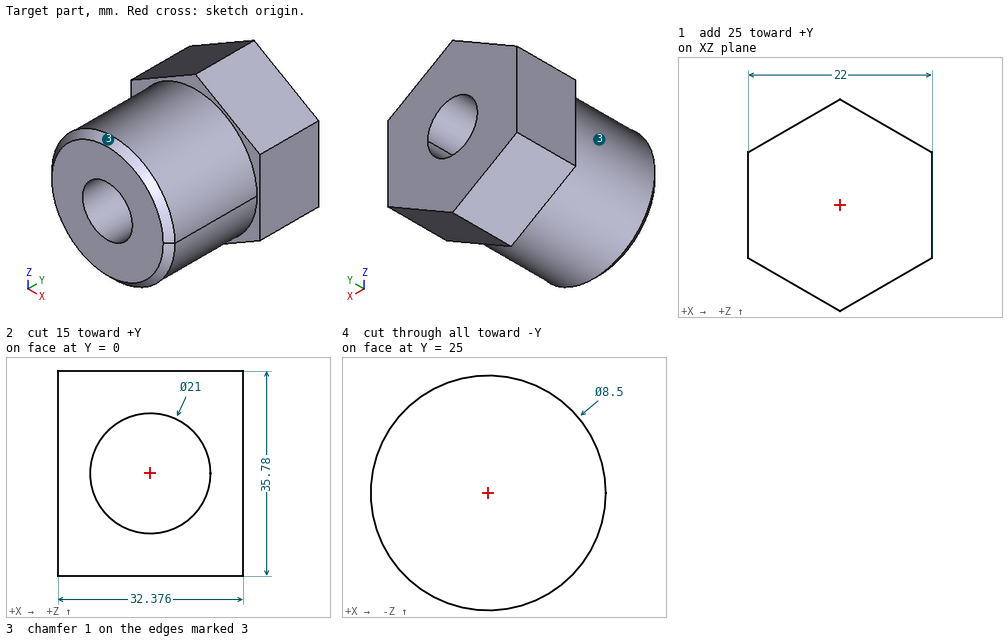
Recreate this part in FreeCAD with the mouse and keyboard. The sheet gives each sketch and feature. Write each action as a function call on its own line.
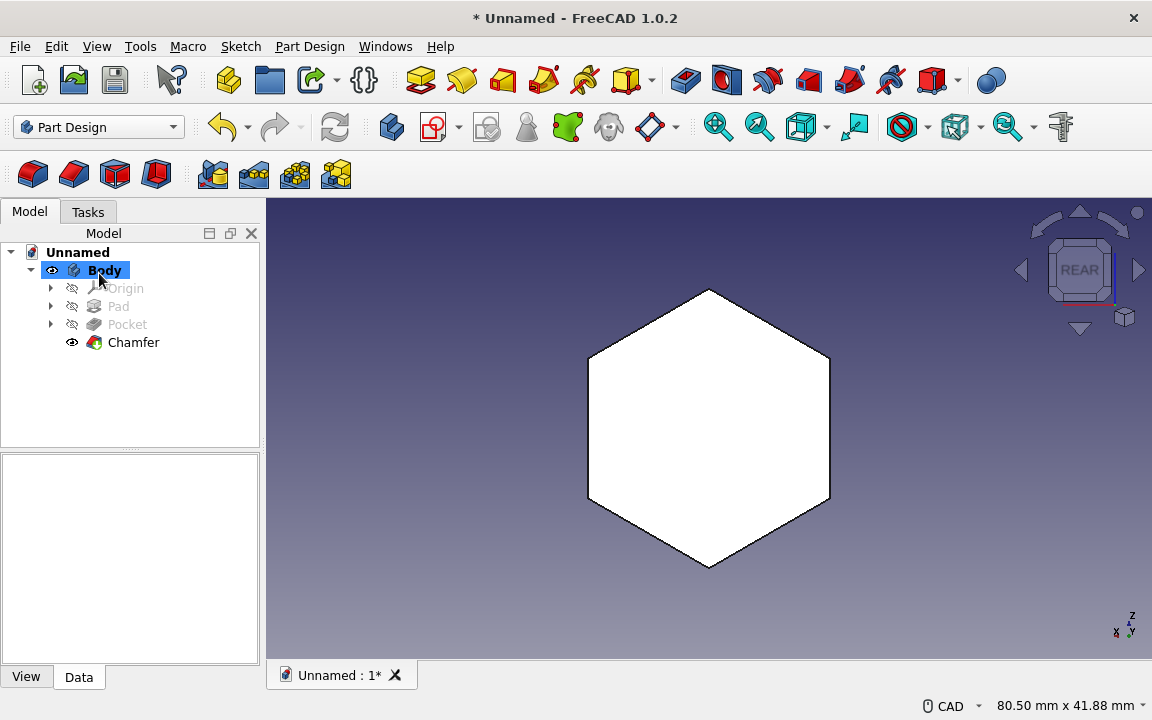
click(709, 428)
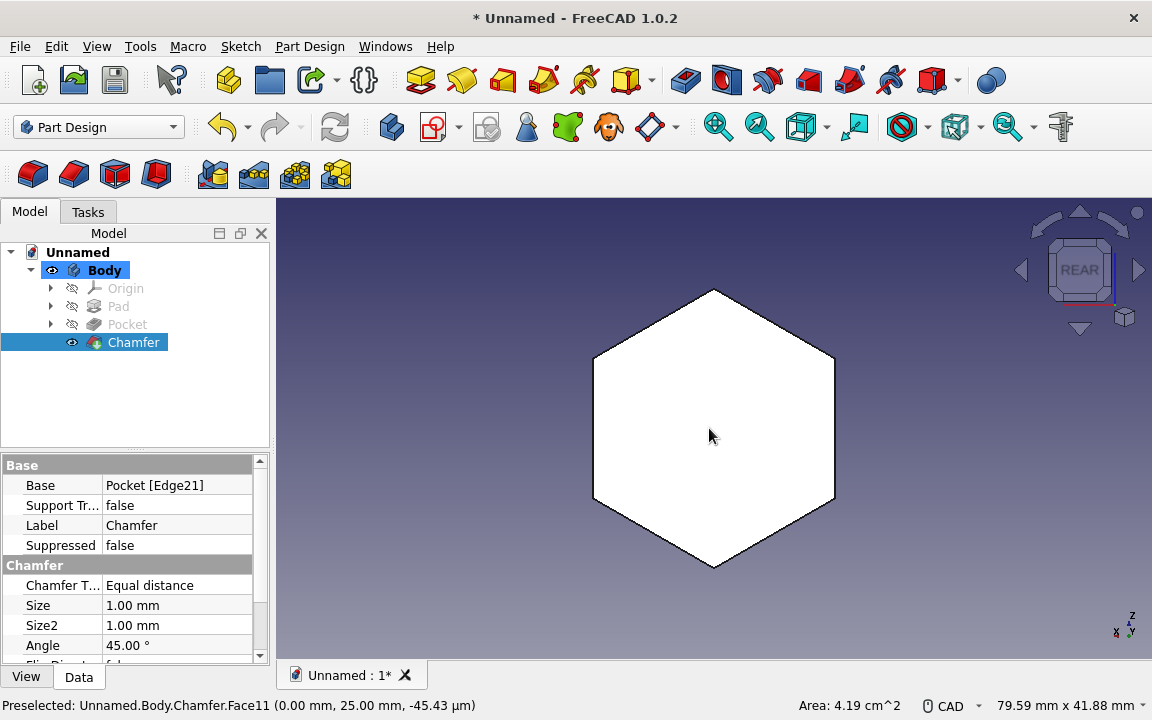
click(432, 128)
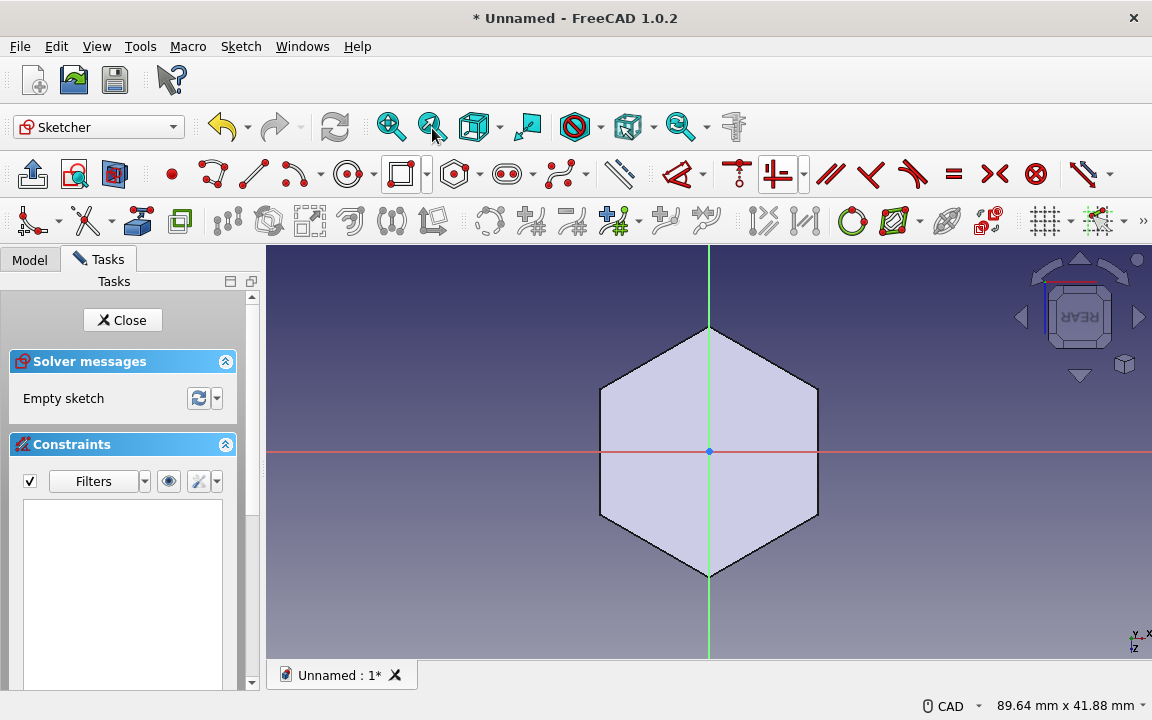
scroll(739, 452, up, 6)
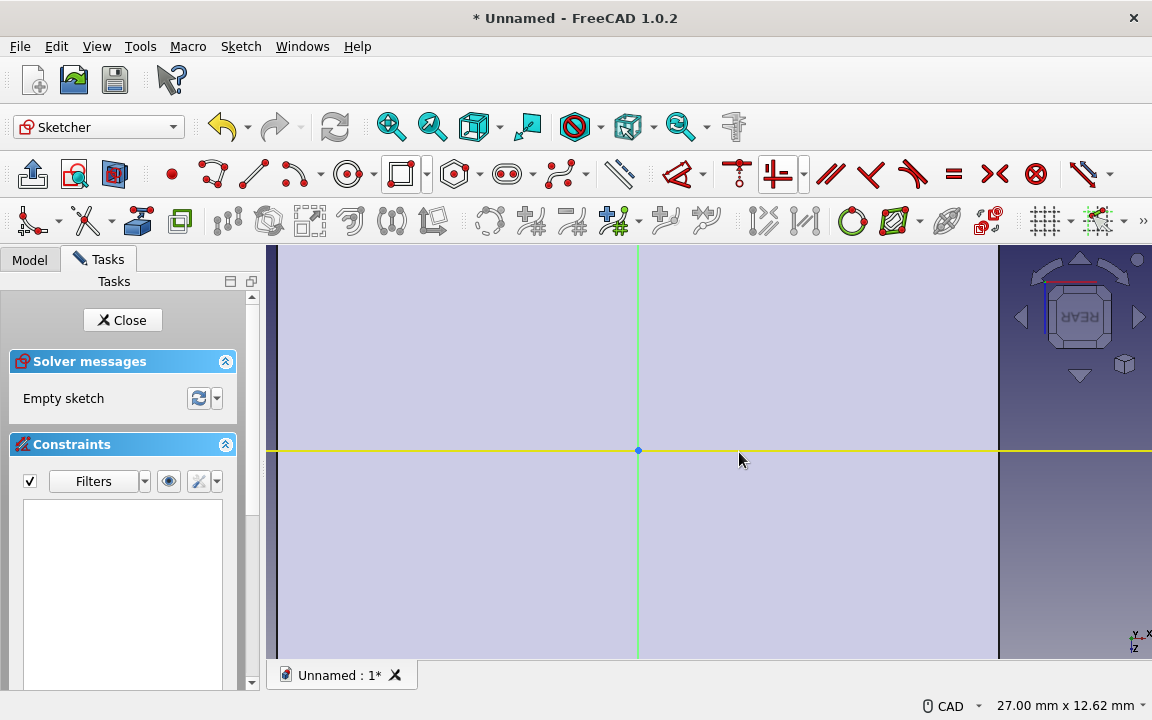
key(g)
key(c)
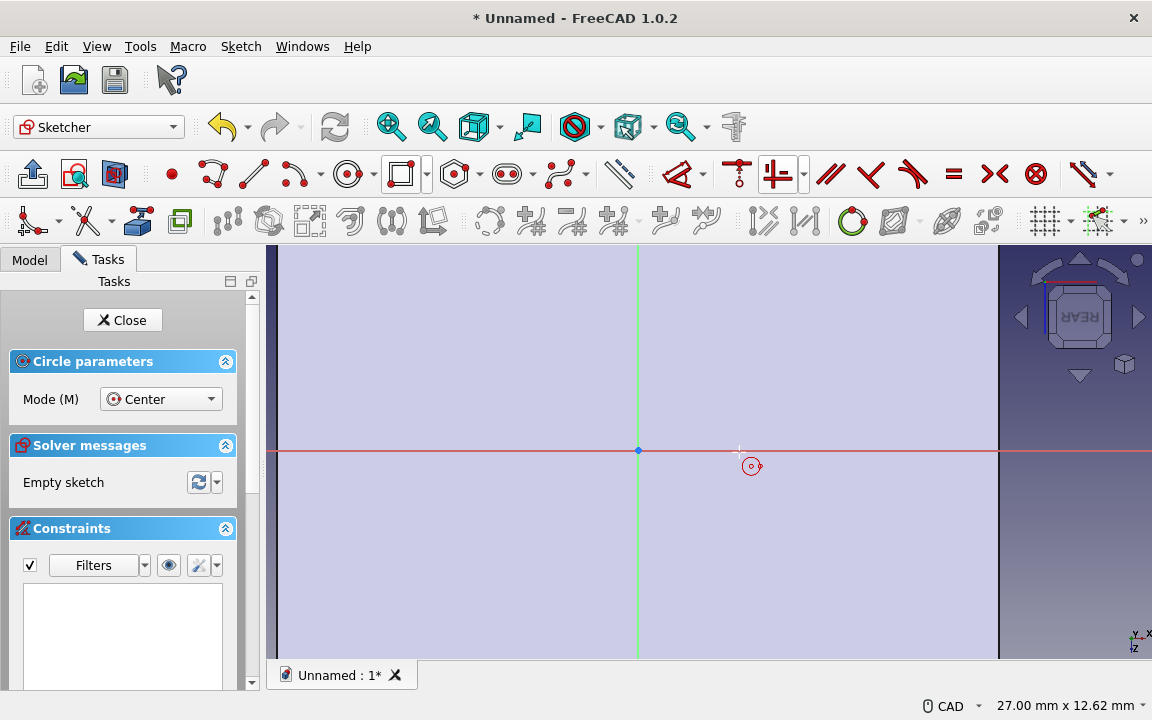
click(638, 451)
move(737, 352)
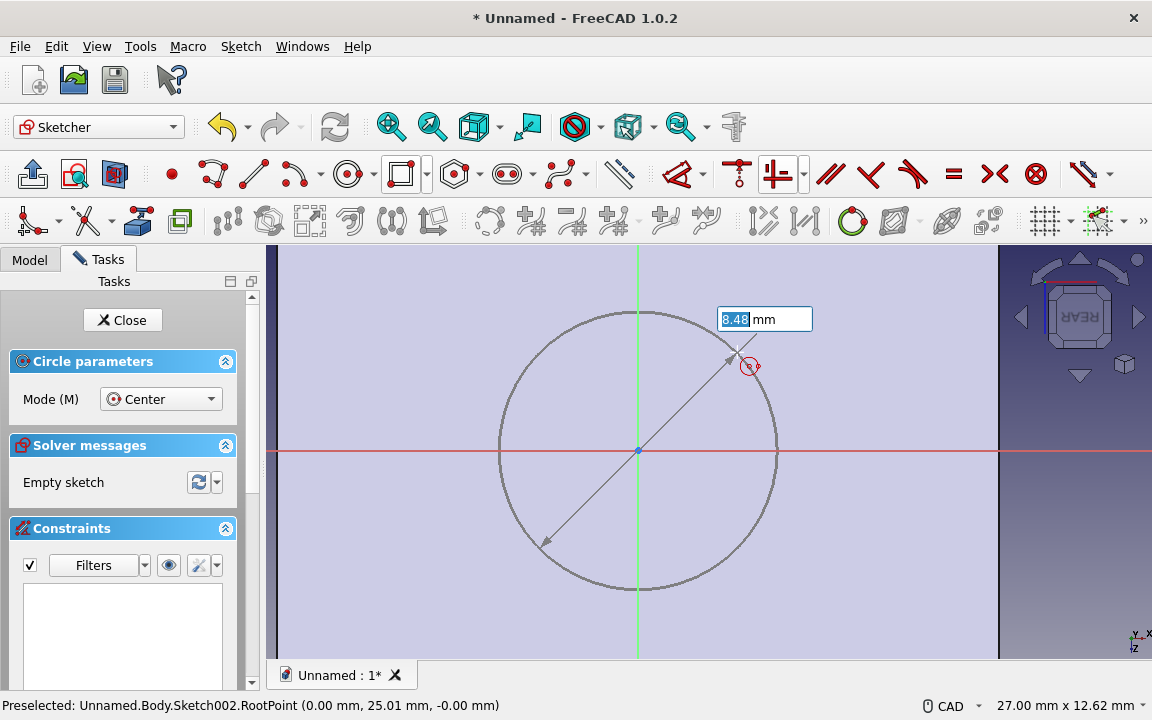
text(8.5)
key(Return)
key(Escape)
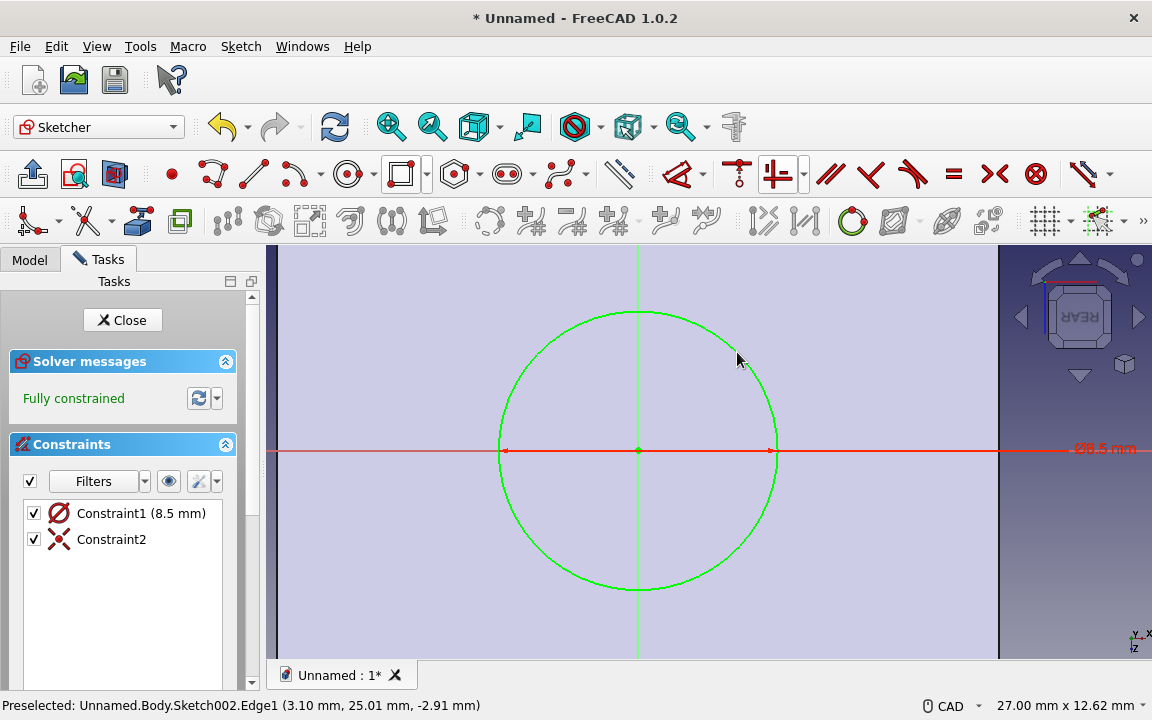
click(123, 320)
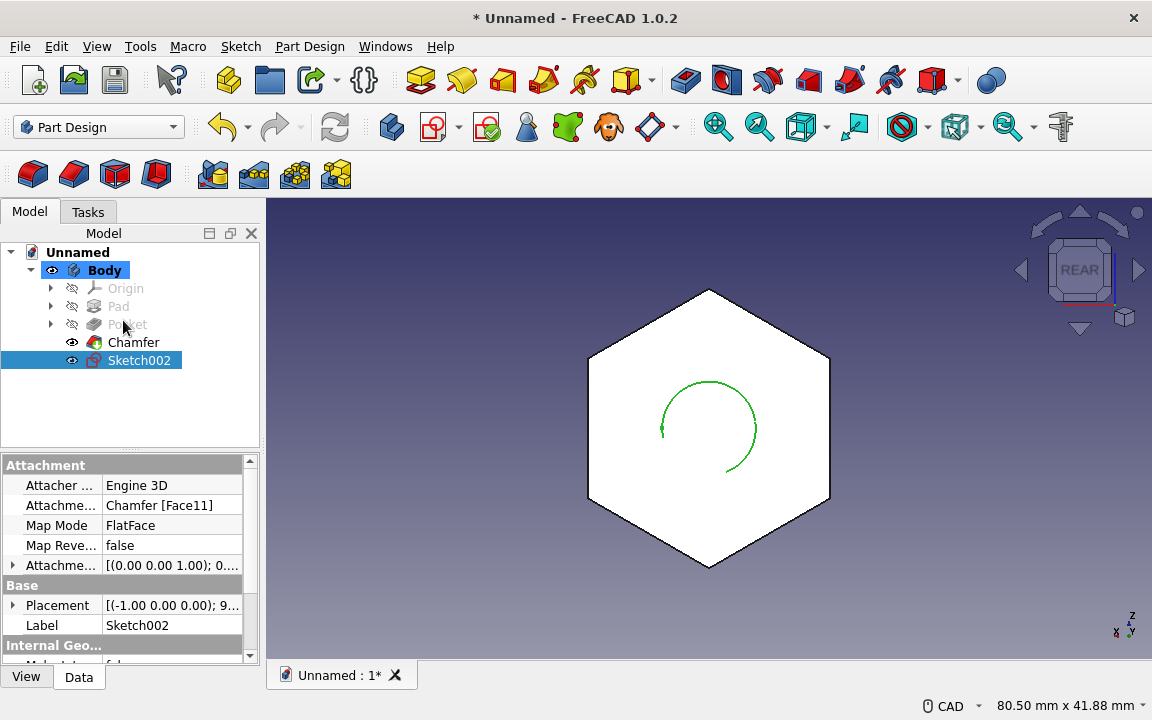
click(686, 80)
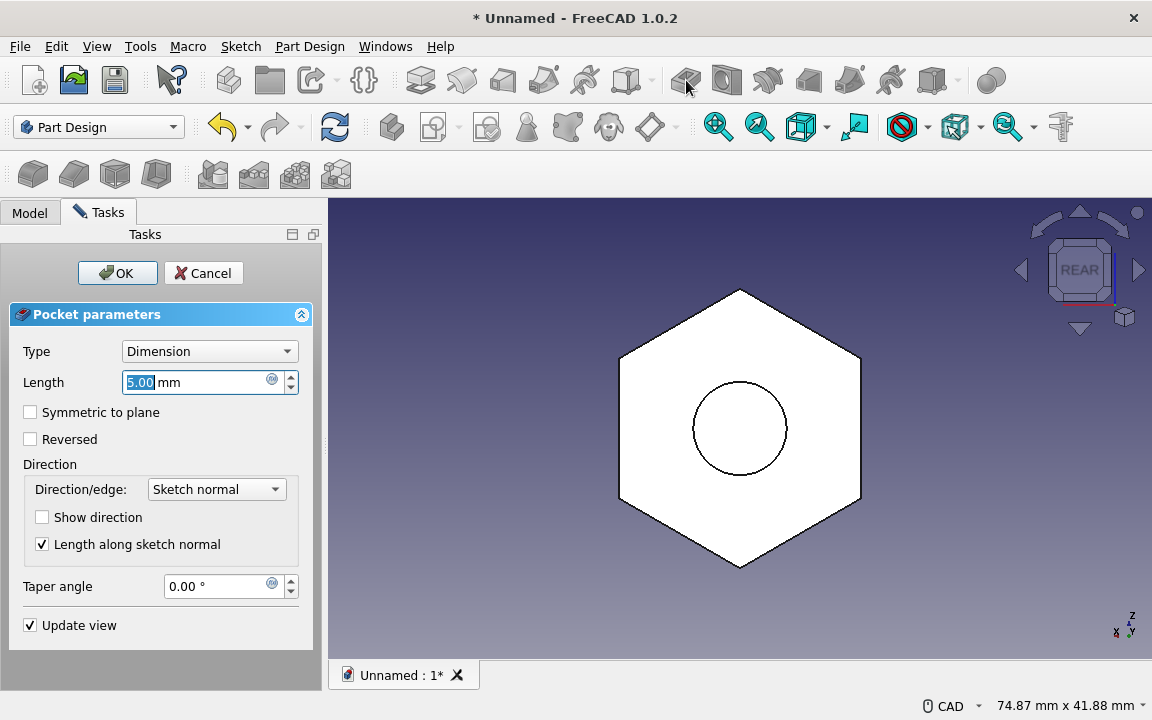
click(210, 352)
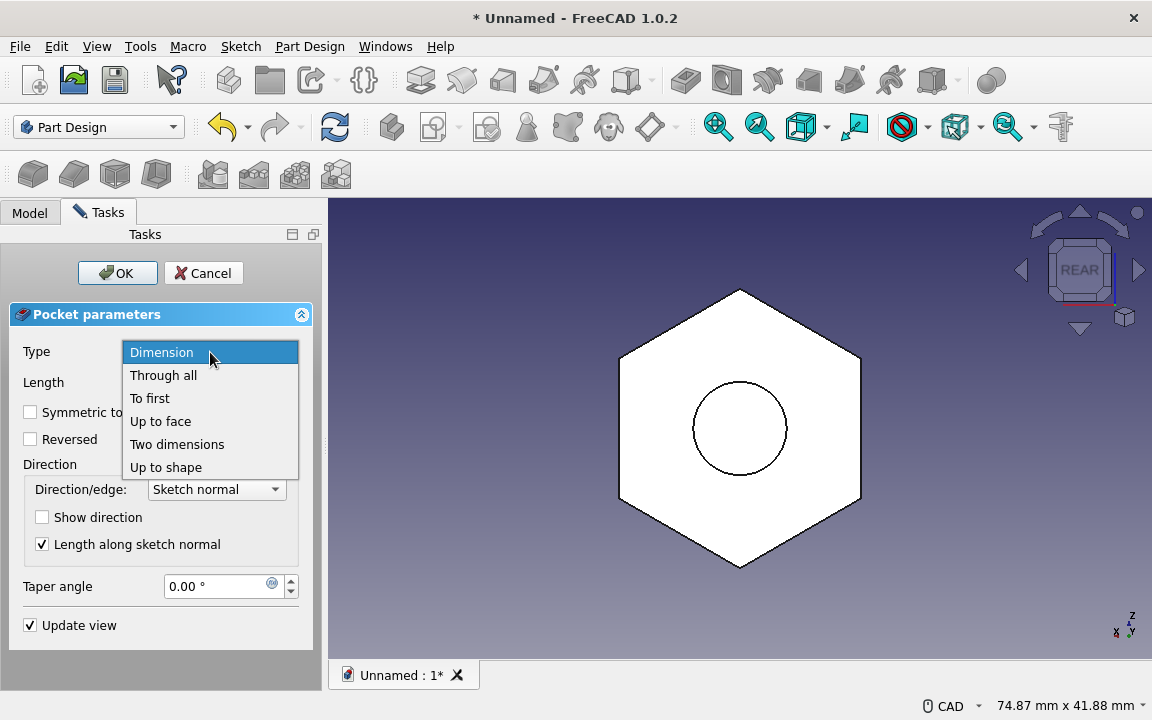
click(208, 376)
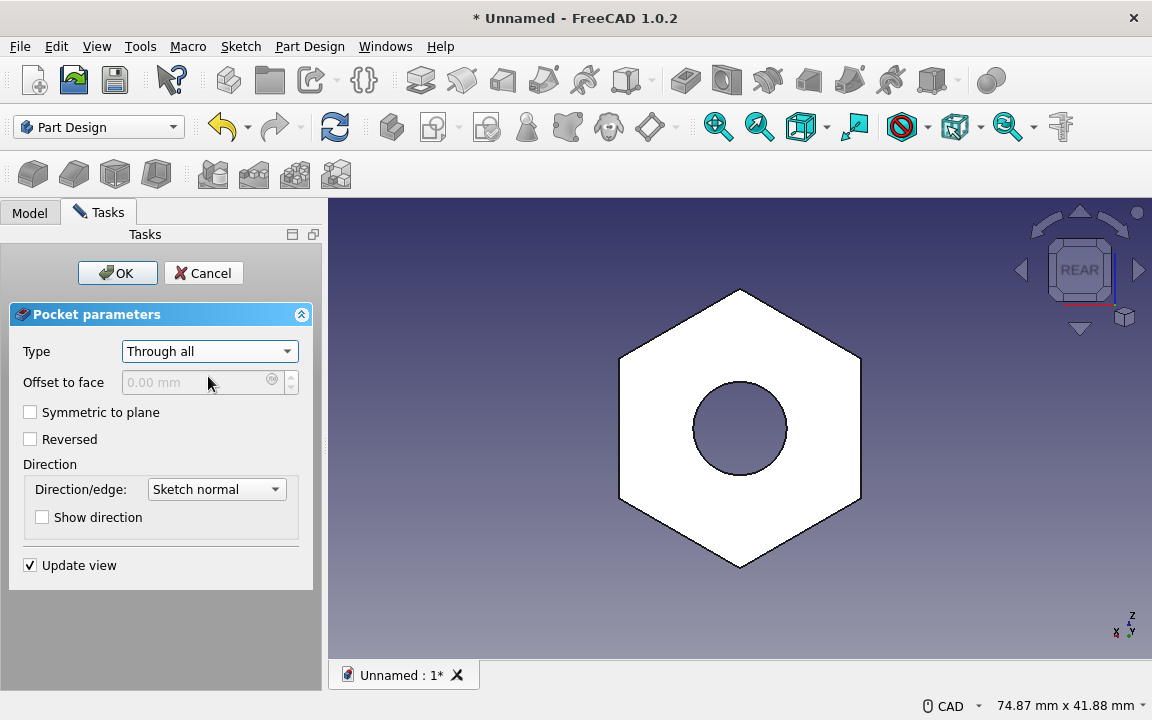
click(118, 273)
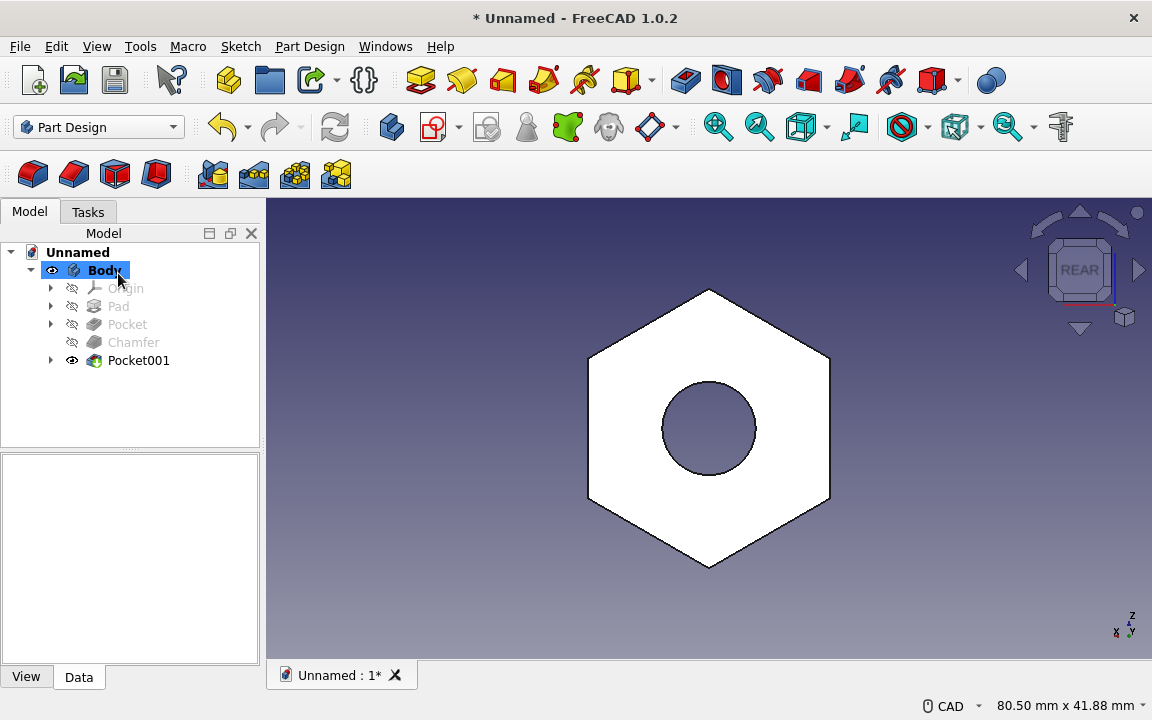
key(0)